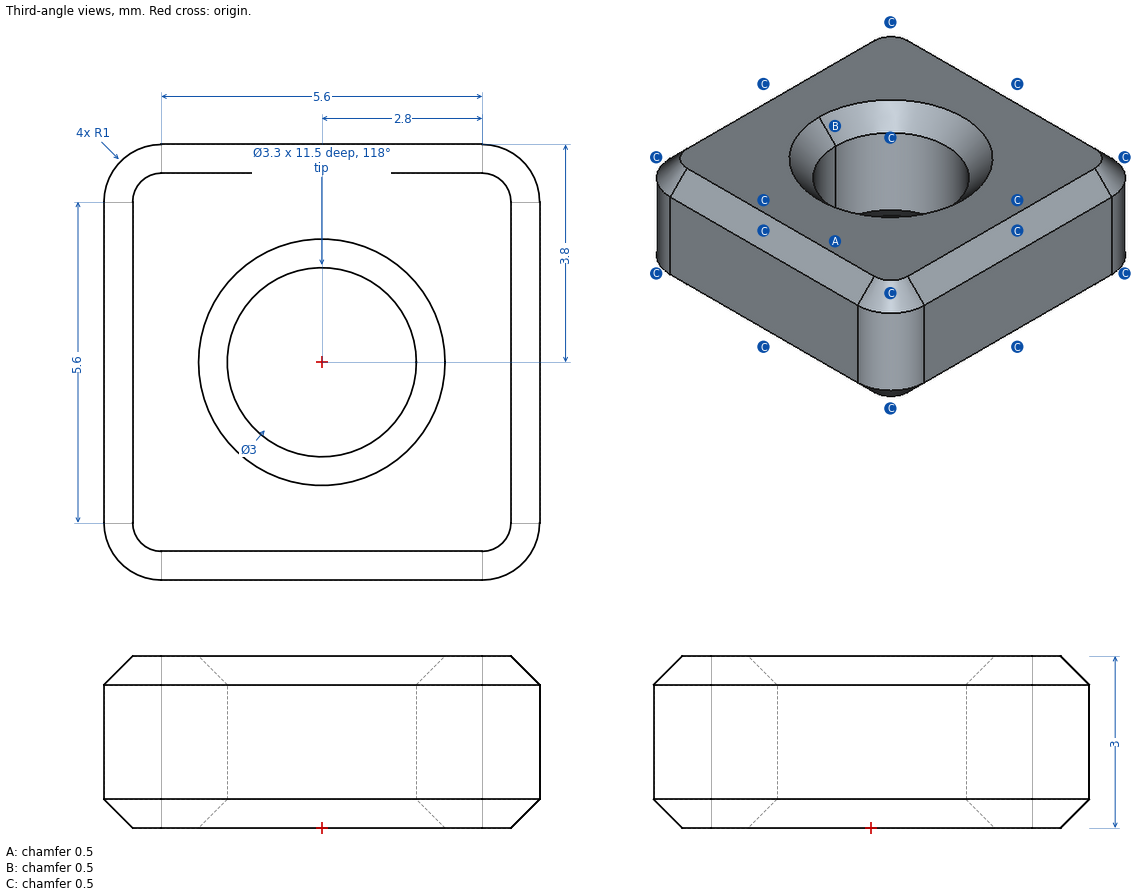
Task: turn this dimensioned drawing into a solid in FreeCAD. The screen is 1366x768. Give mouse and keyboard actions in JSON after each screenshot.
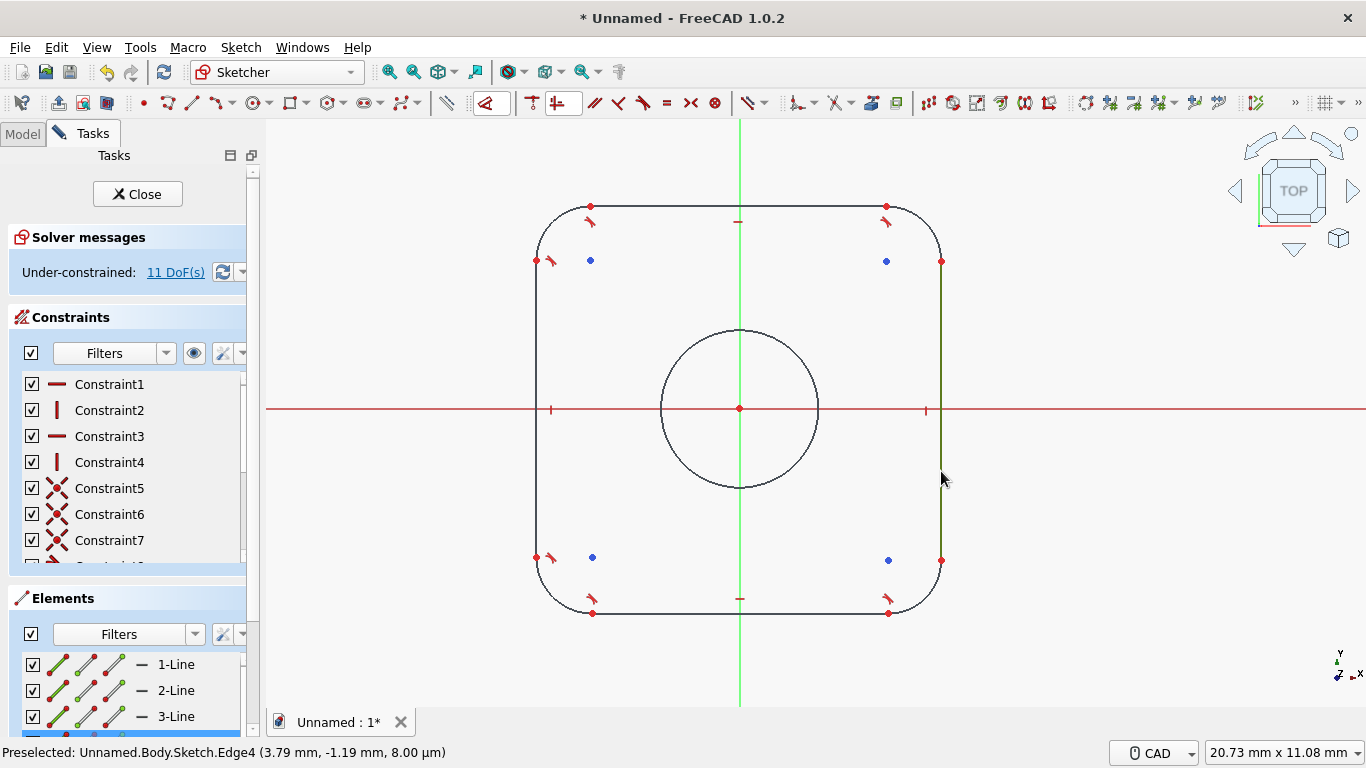
{"action": "left_click", "coordinate": [912, 608]}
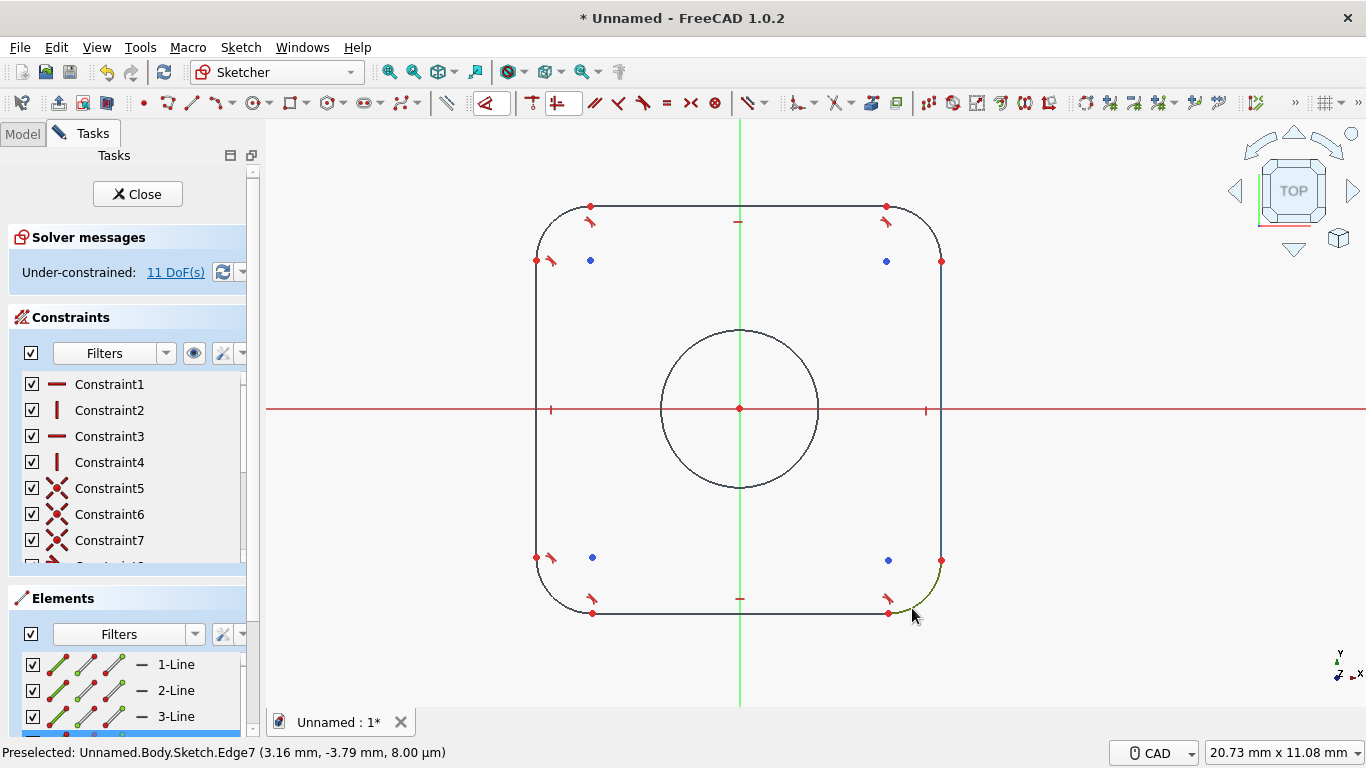
{"action": "left_click", "coordinate": [644, 104]}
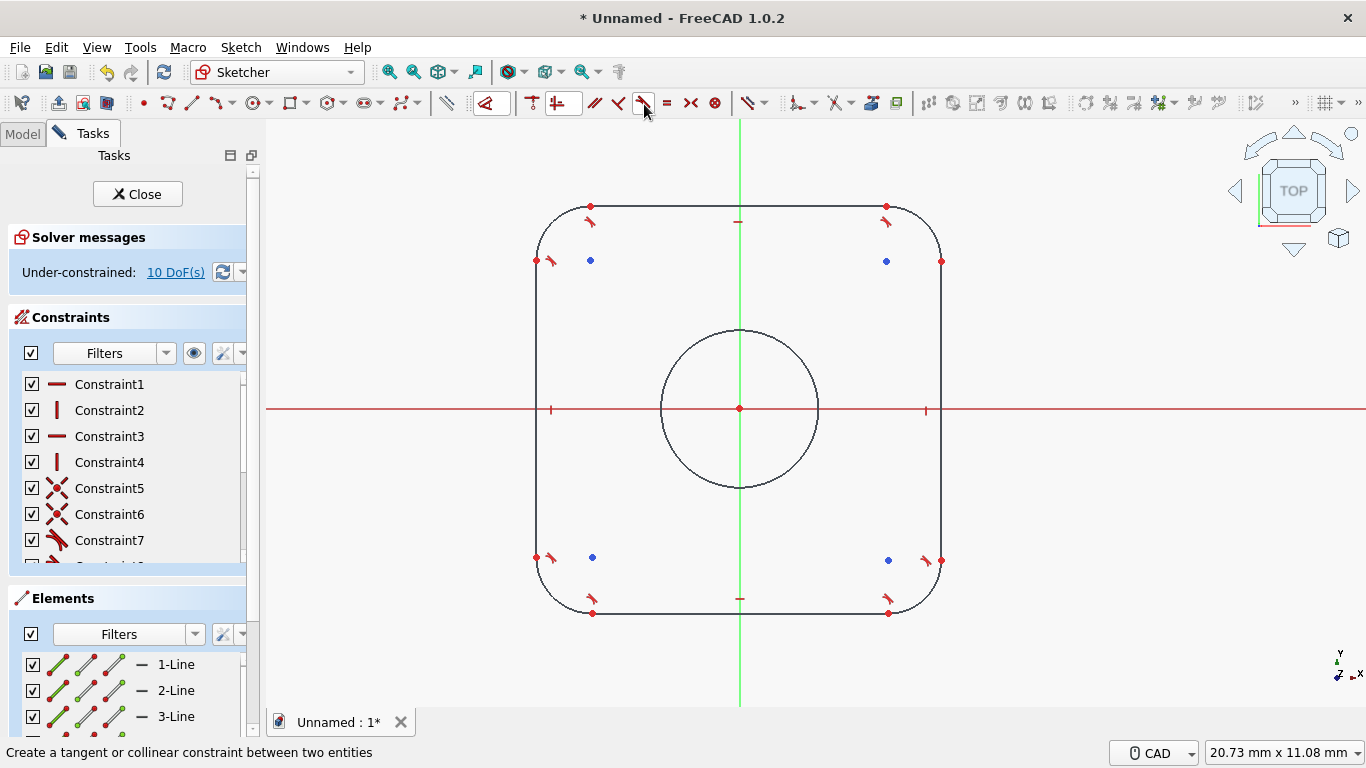
{"action": "left_click", "coordinate": [941, 471]}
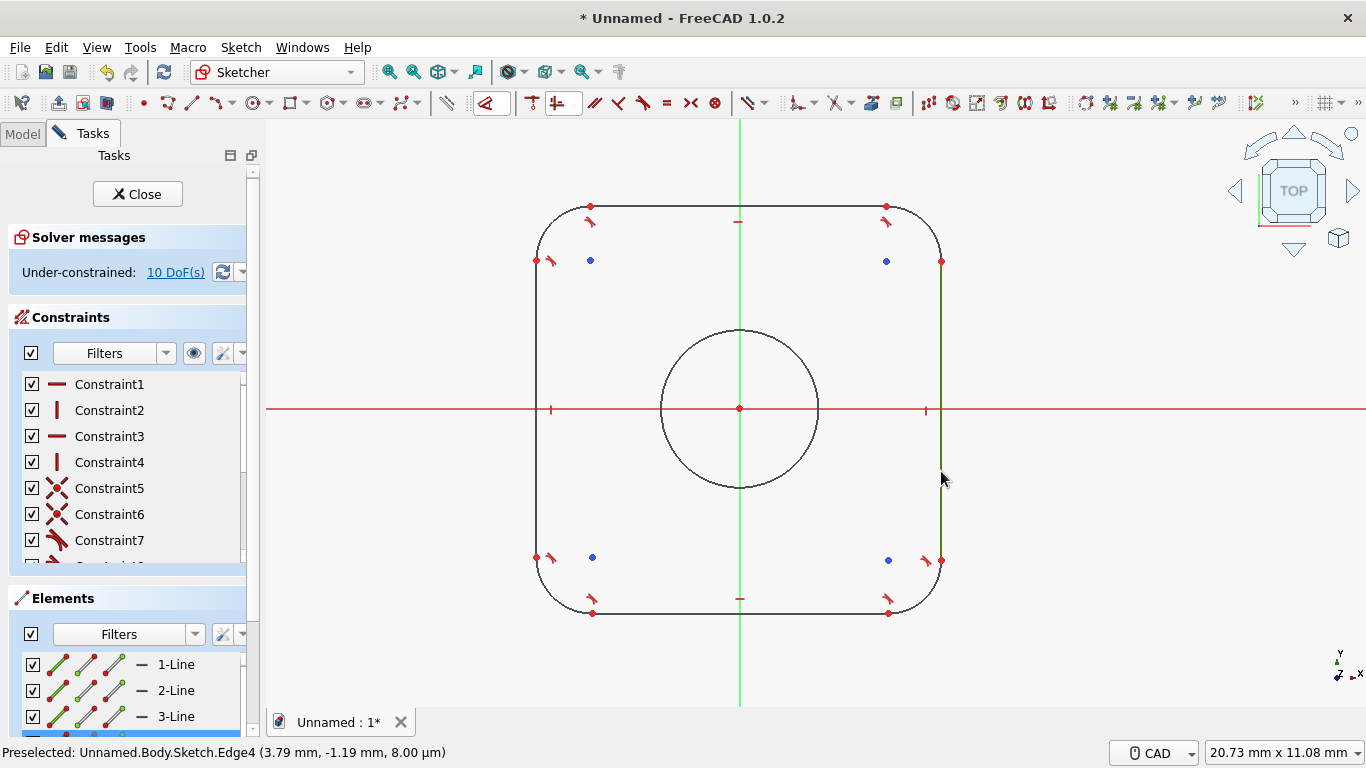
{"action": "left_click", "coordinate": [935, 236]}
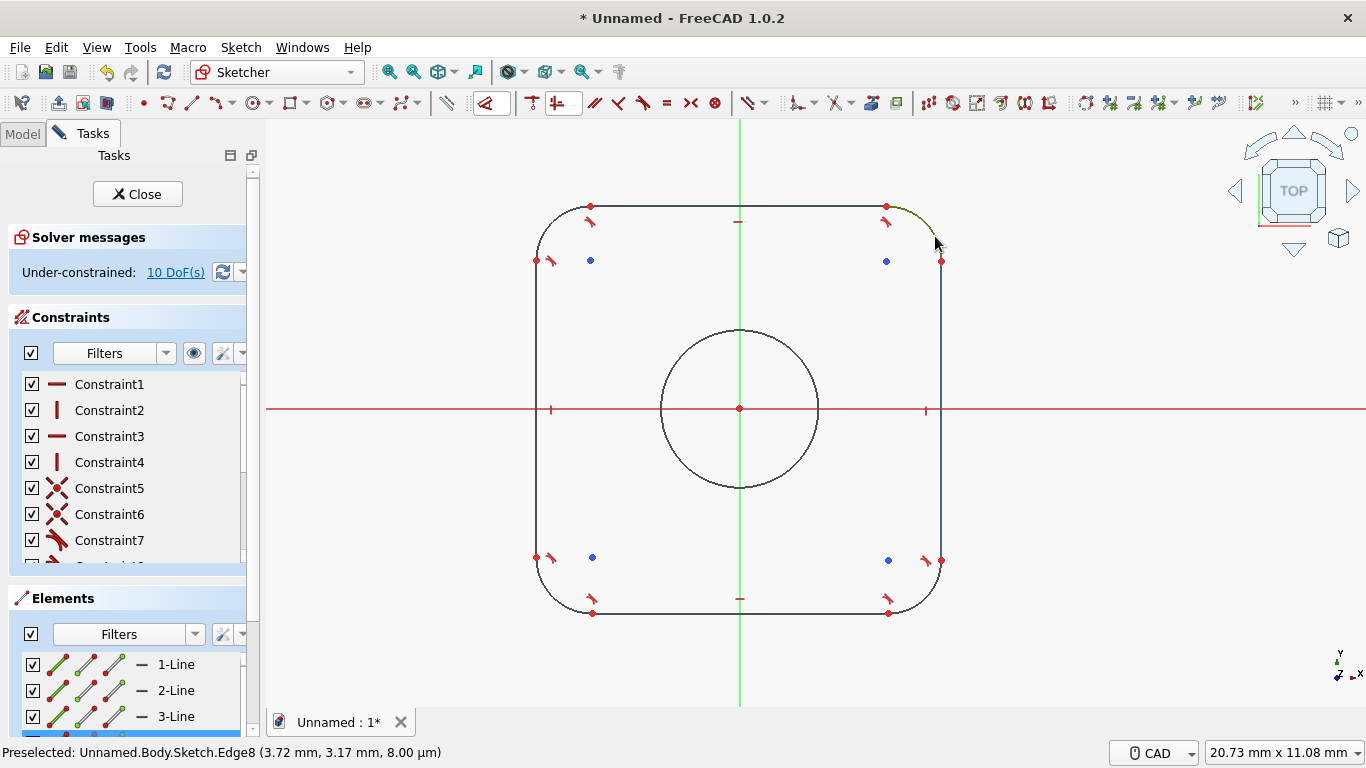
{"action": "key", "text": "t"}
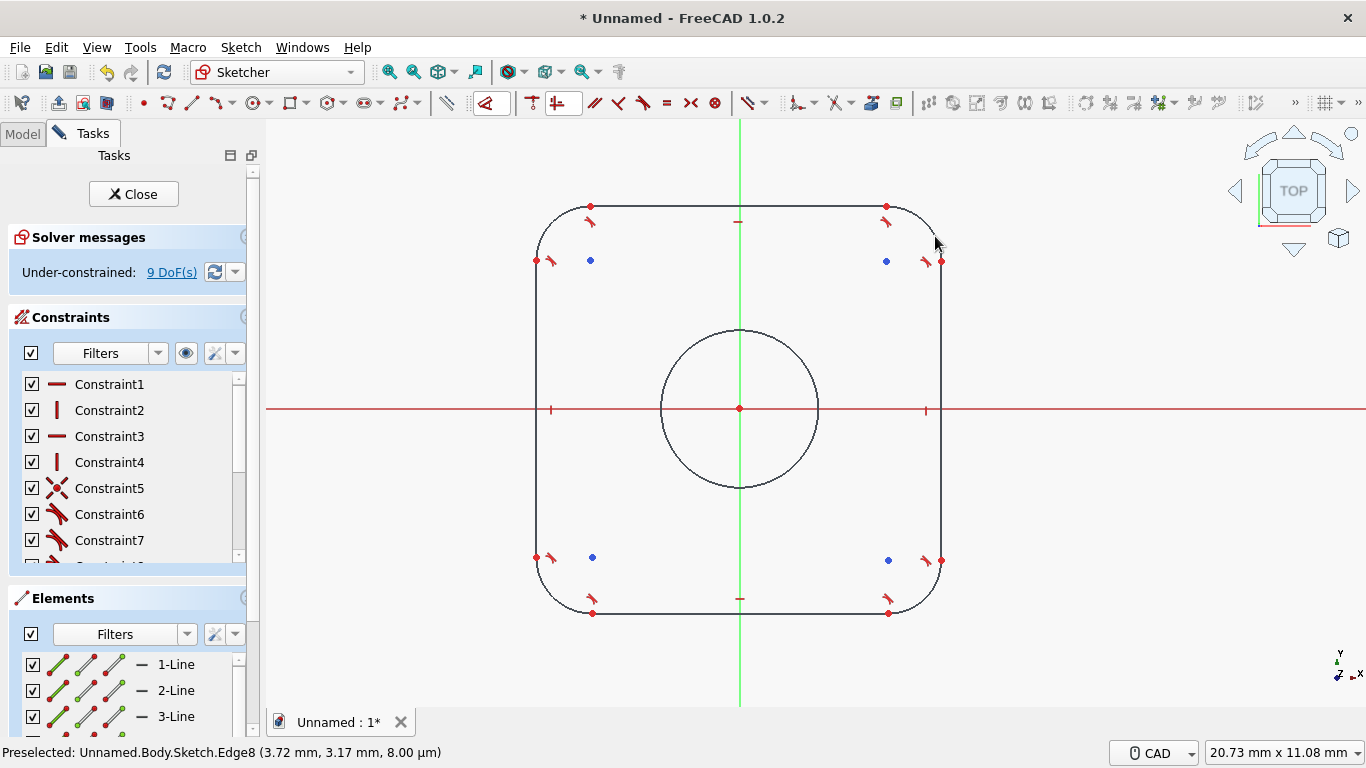
{"action": "left_click", "coordinate": [566, 212]}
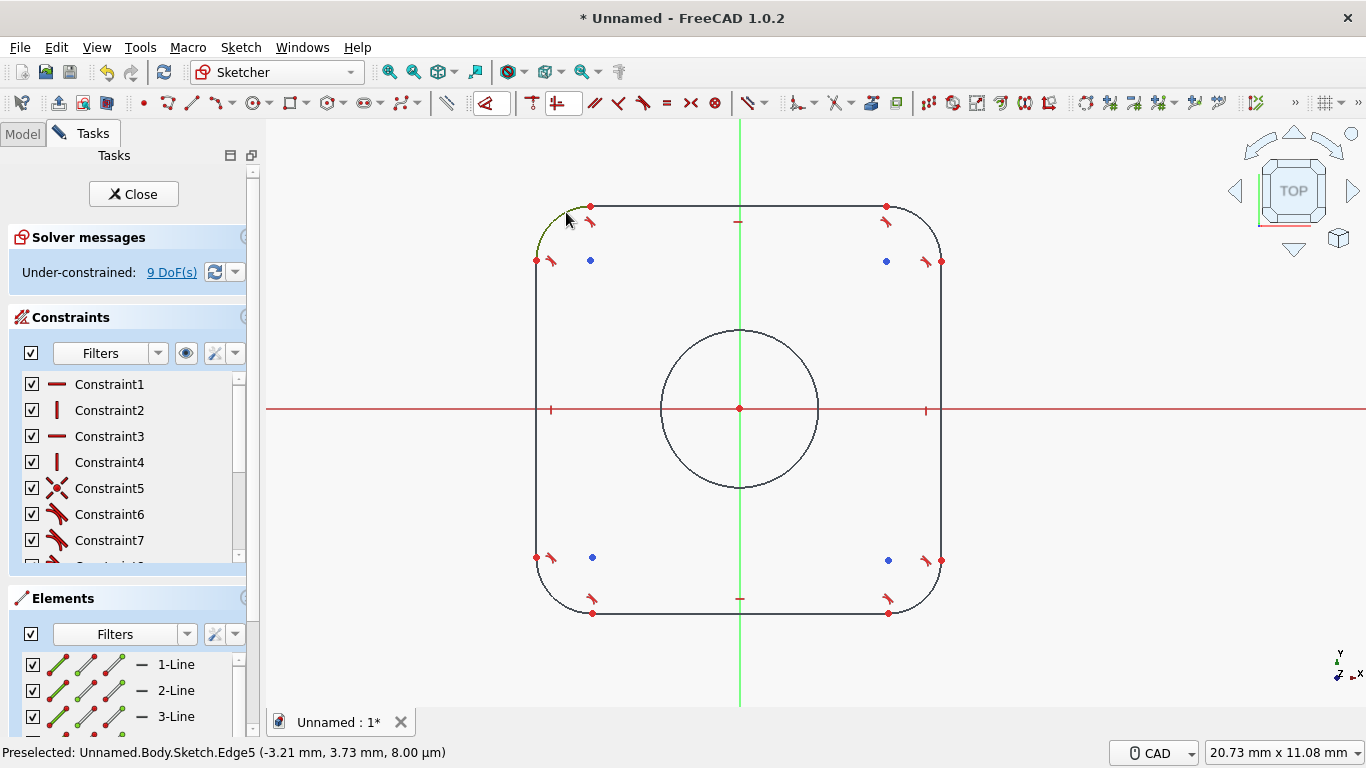
{"action": "left_click", "coordinate": [543, 583]}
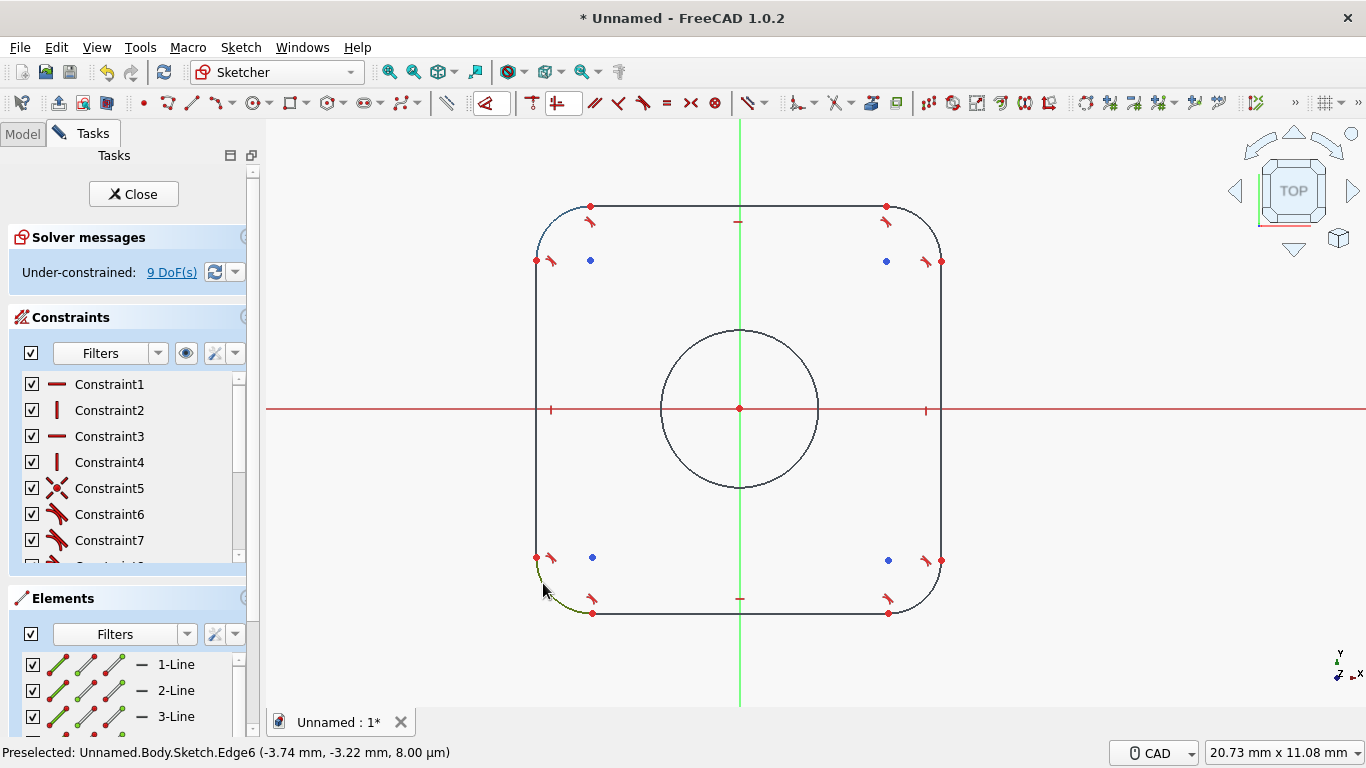
{"action": "left_click", "coordinate": [912, 608]}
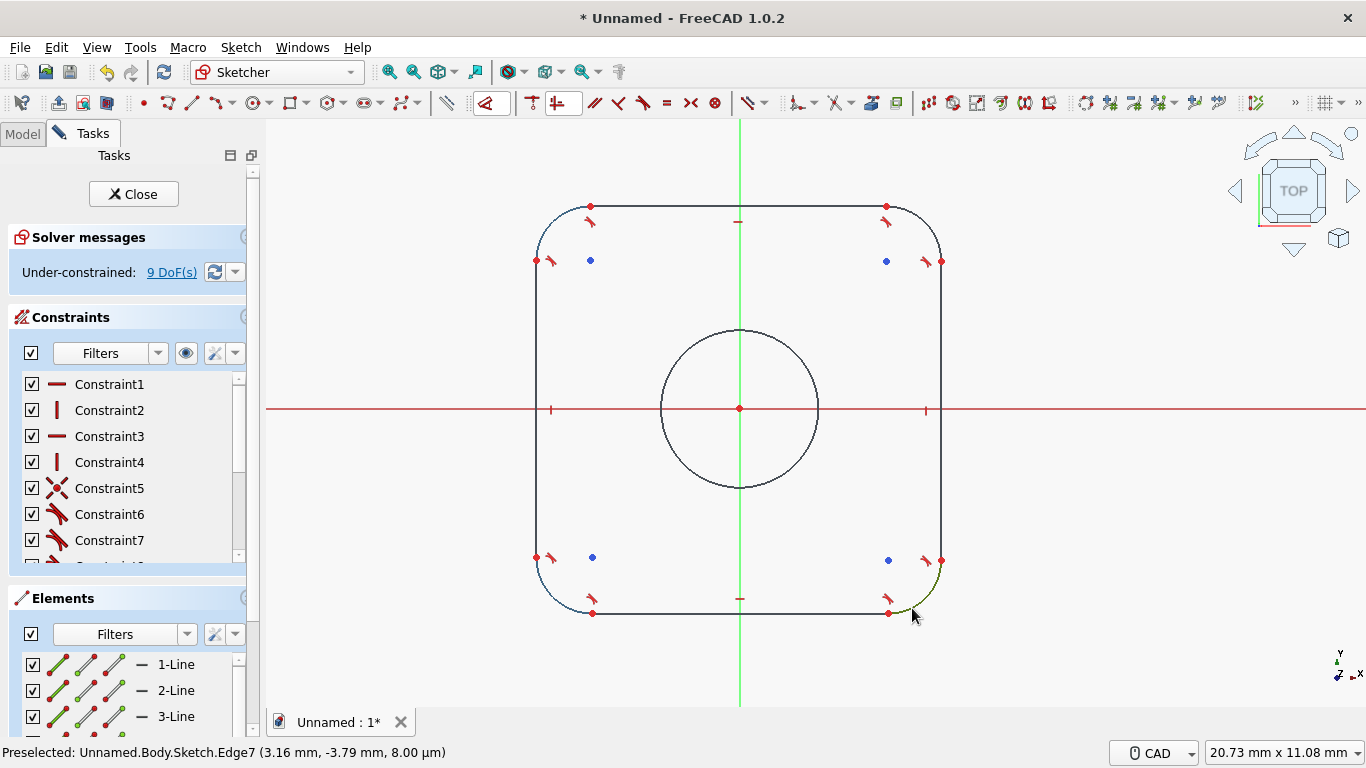
{"action": "left_click", "coordinate": [935, 236]}